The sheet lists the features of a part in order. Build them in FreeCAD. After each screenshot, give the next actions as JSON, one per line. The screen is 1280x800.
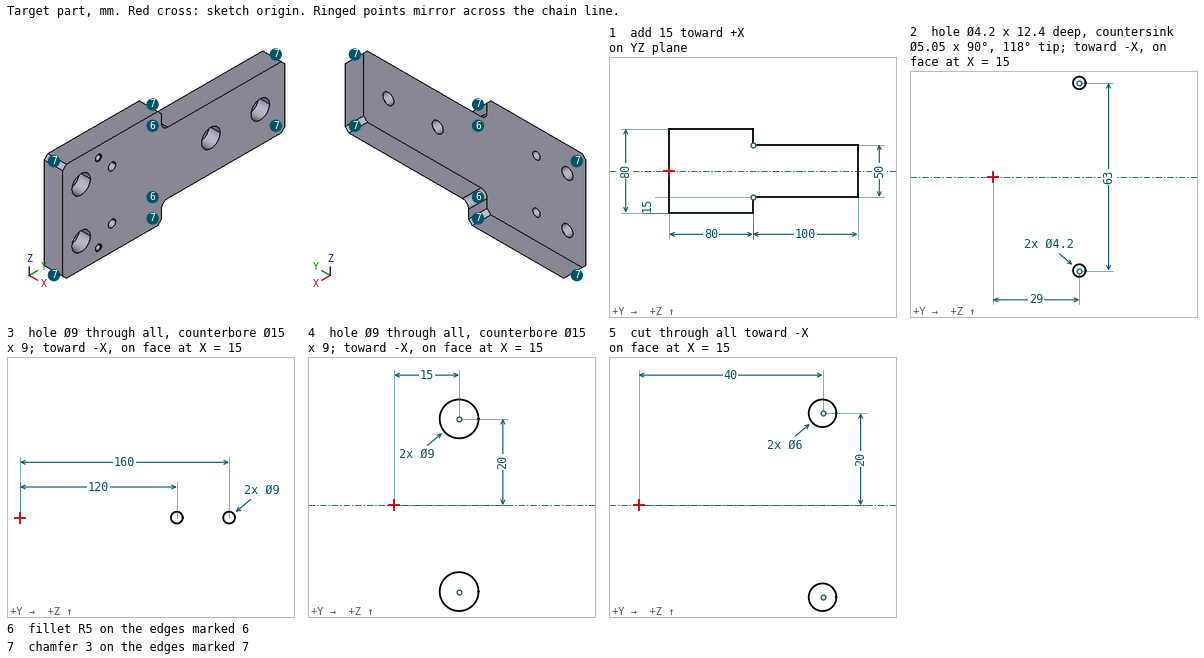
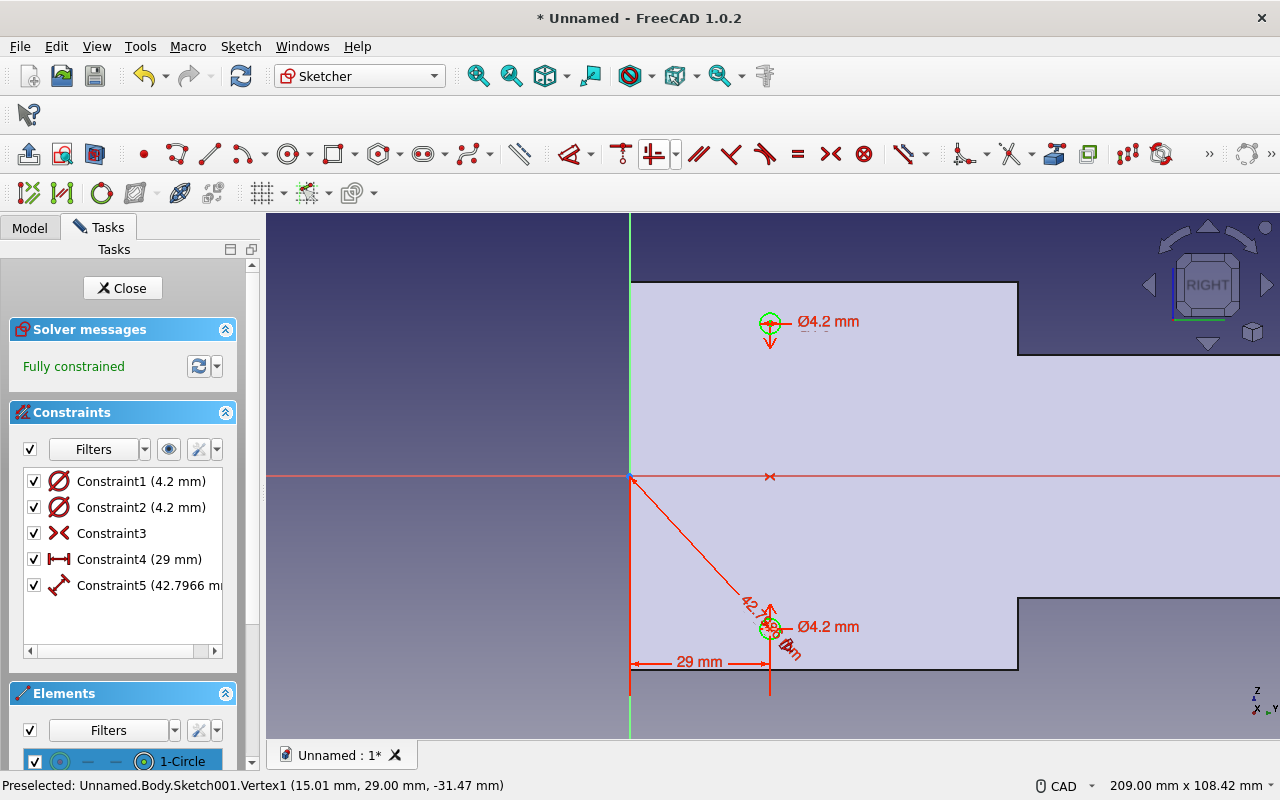
{"action": "left_click", "coordinate": [770, 324]}
{"action": "left_click", "coordinate": [804, 406]}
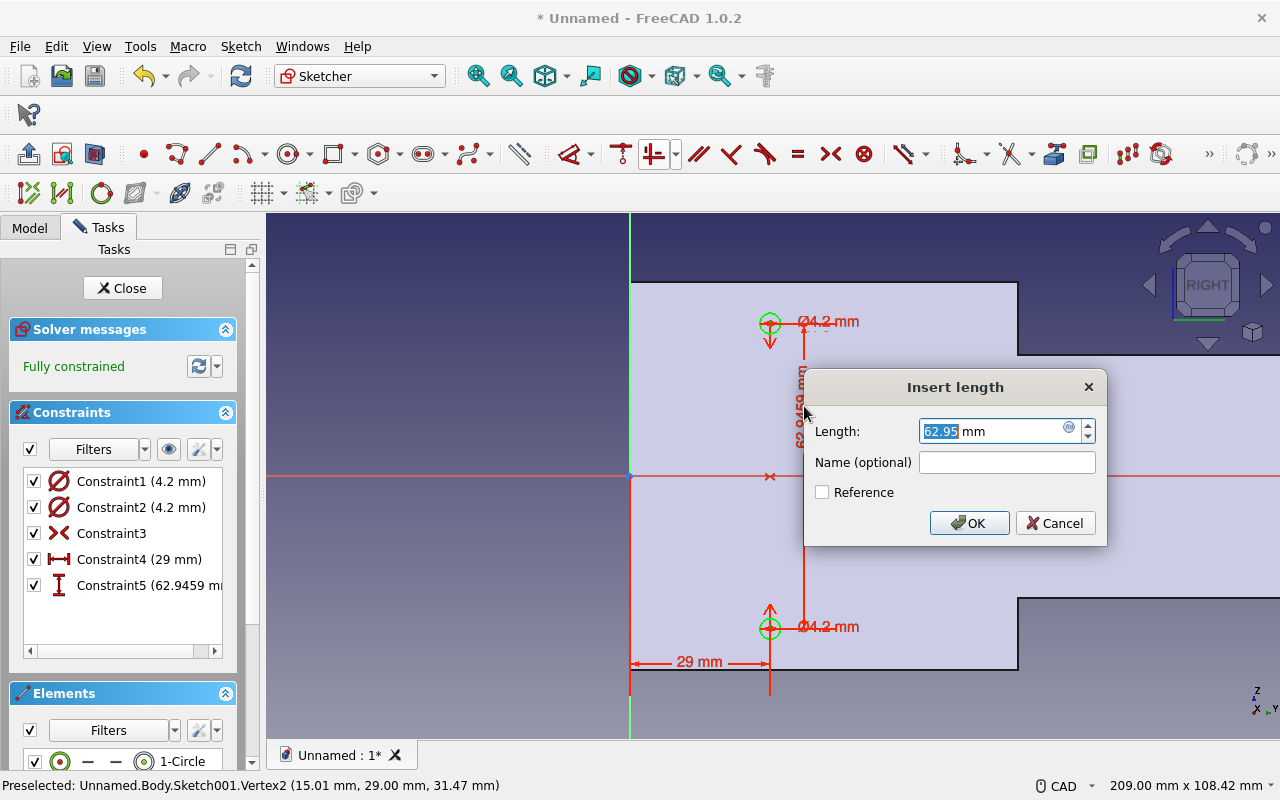
{"action": "type", "text": "63"}
{"action": "key", "text": "Return"}
{"action": "key", "text": "Escape"}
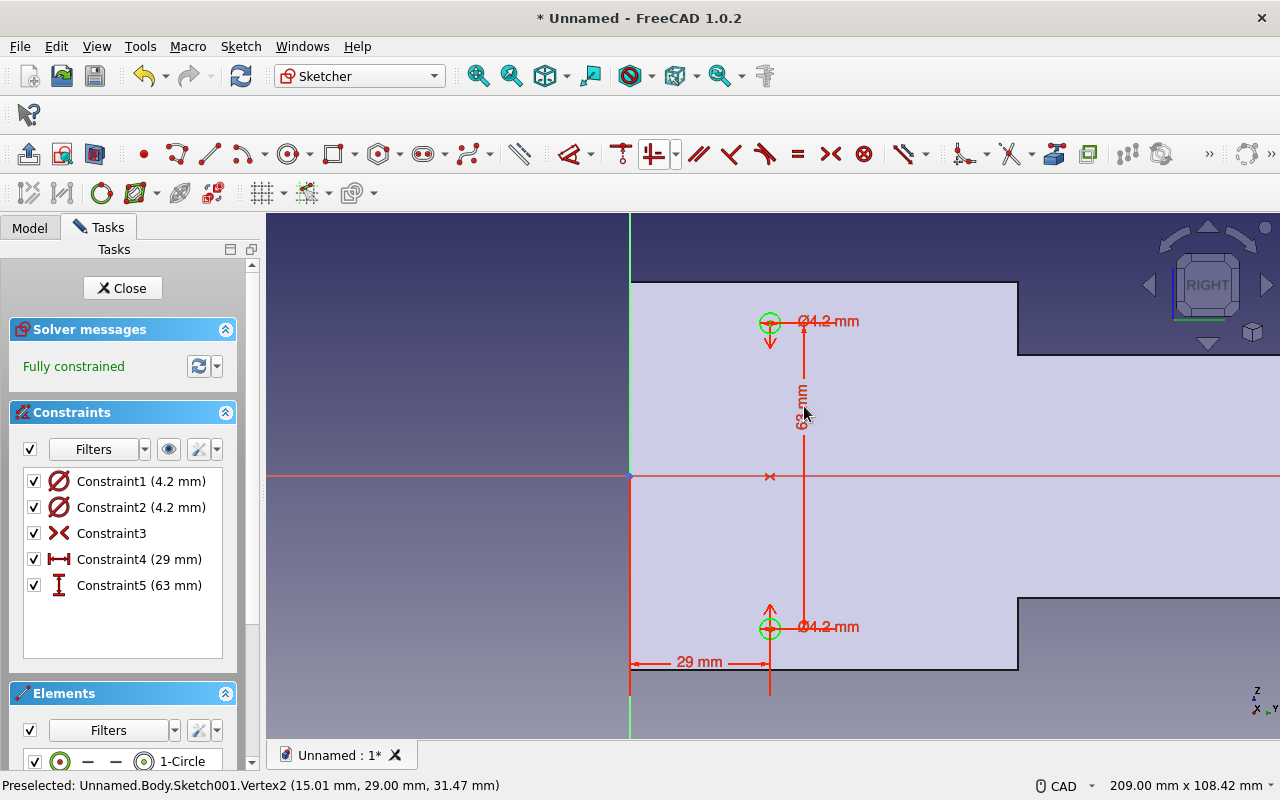
{"action": "left_click", "coordinate": [123, 288]}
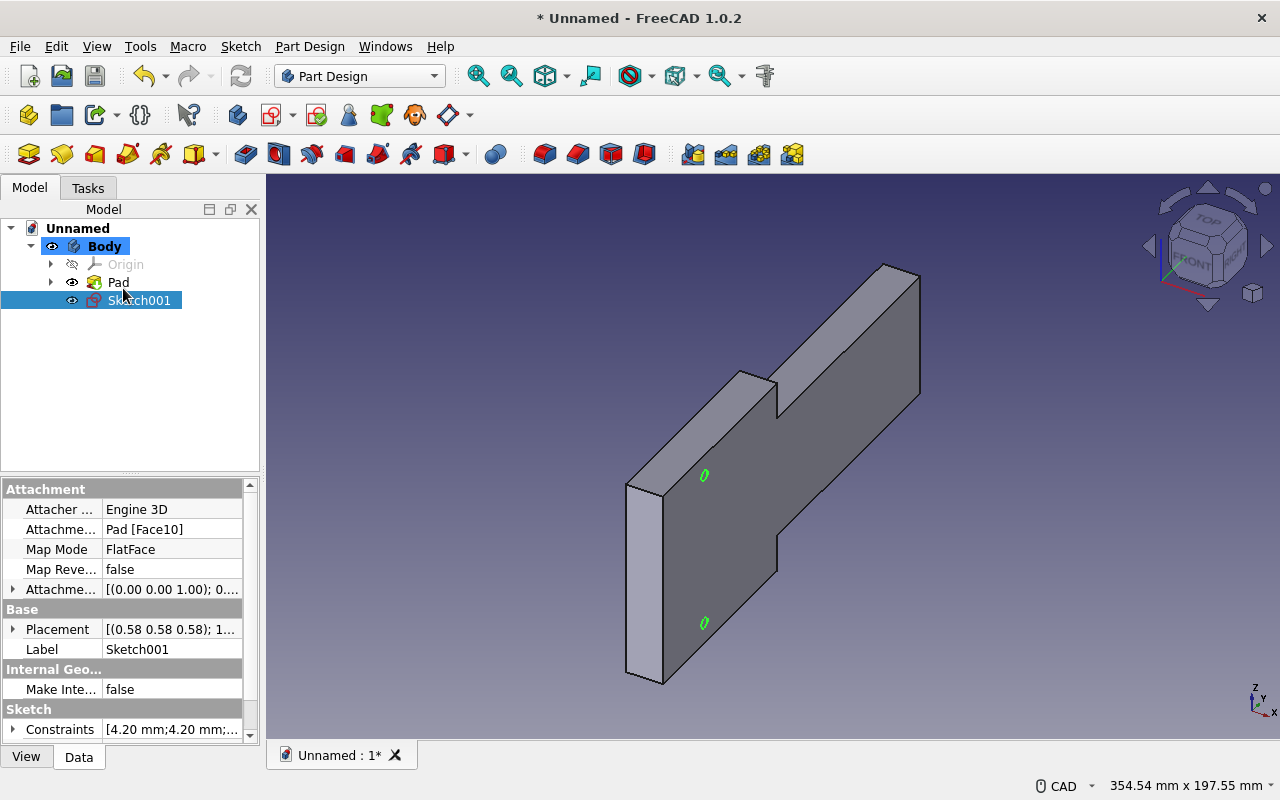
{"action": "left_click", "coordinate": [279, 154]}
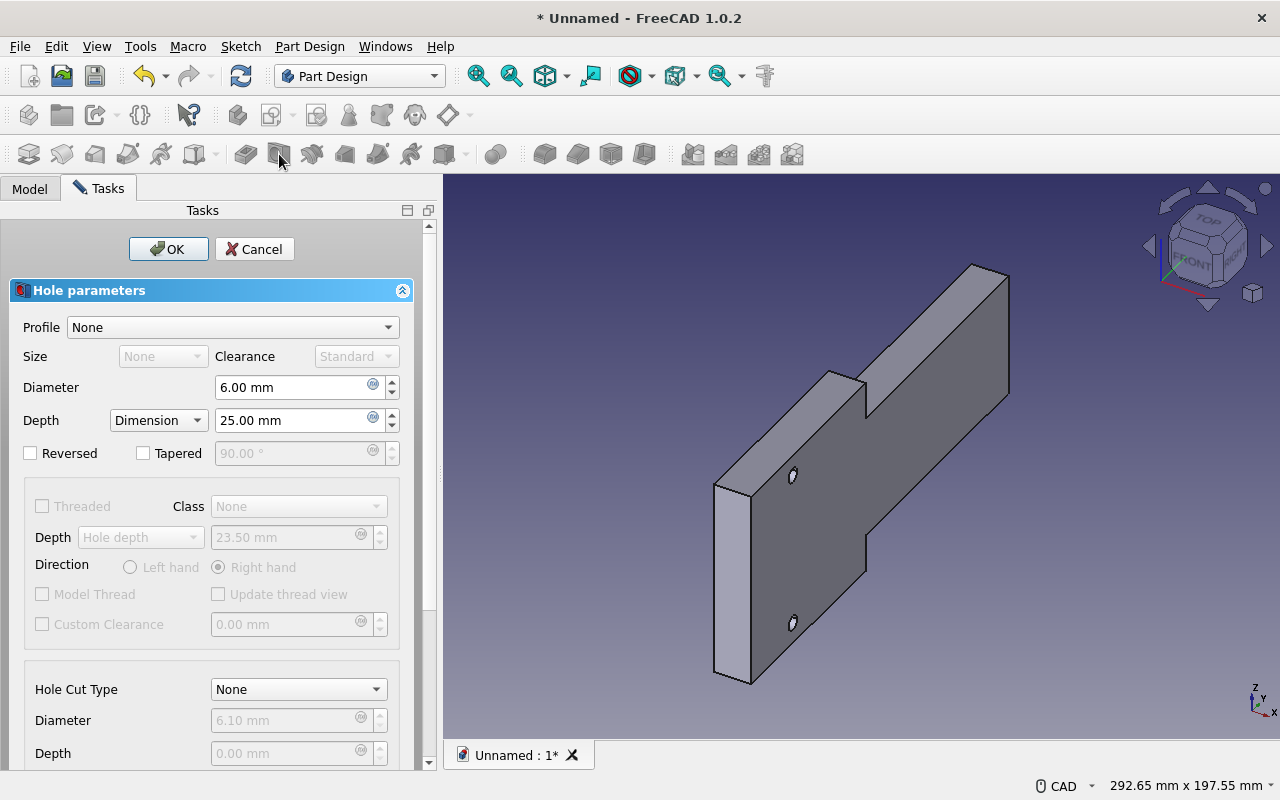
{"action": "triple_click", "coordinate": [300, 388]}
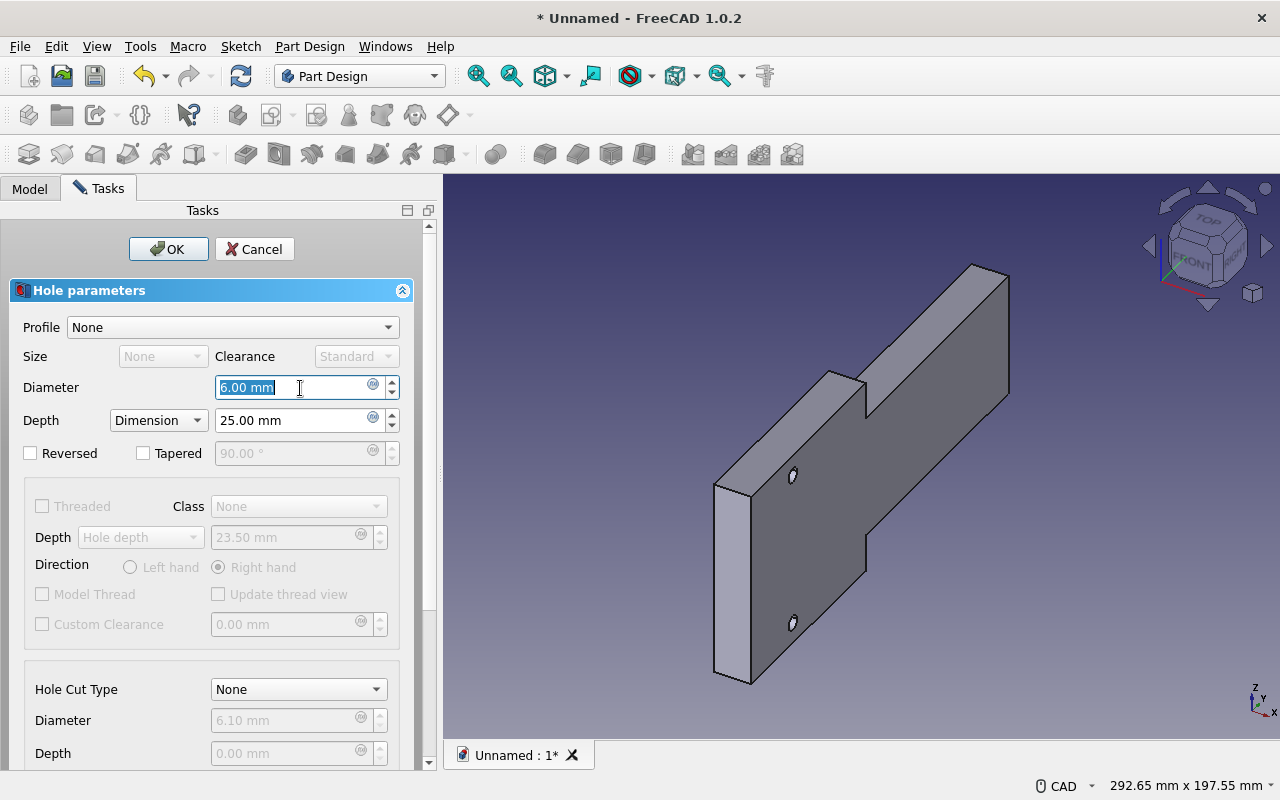
{"action": "type", "text": "4.2"}
{"action": "key", "text": "Tab"}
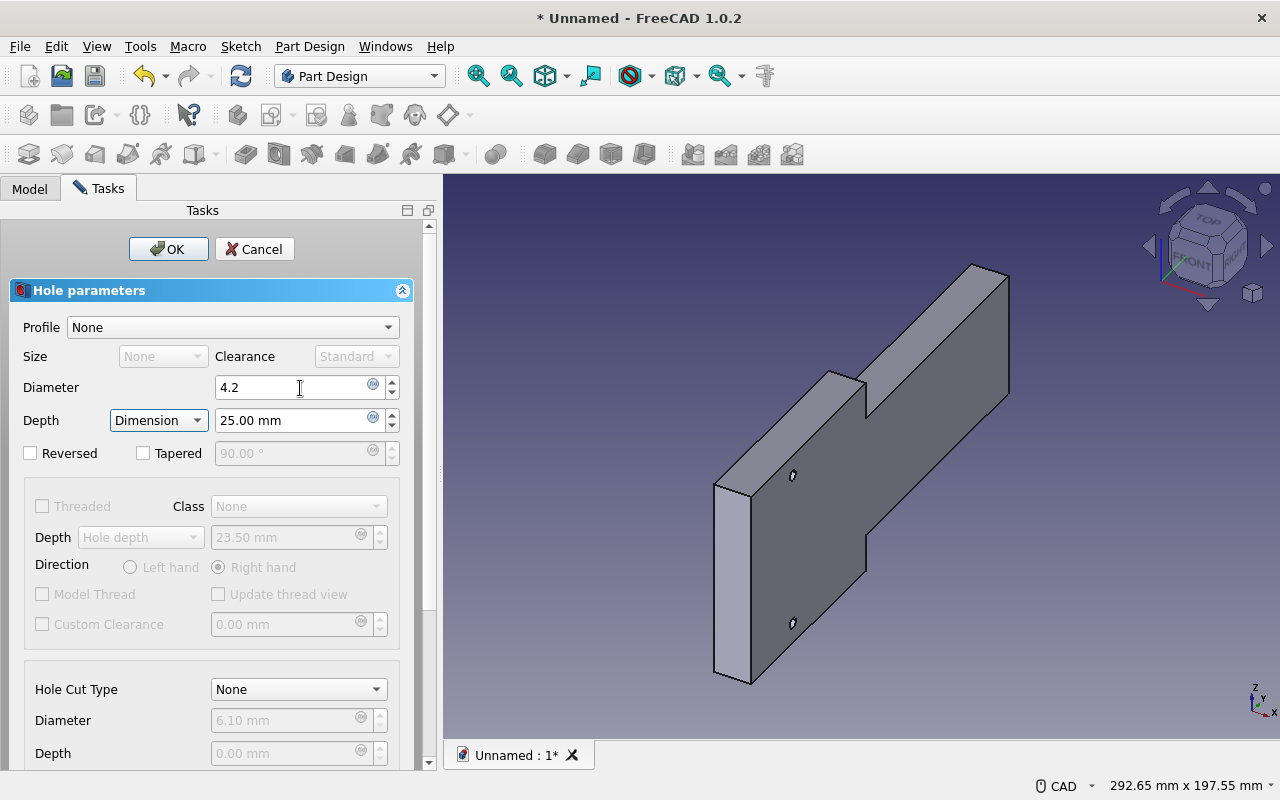
{"action": "triple_click", "coordinate": [300, 420]}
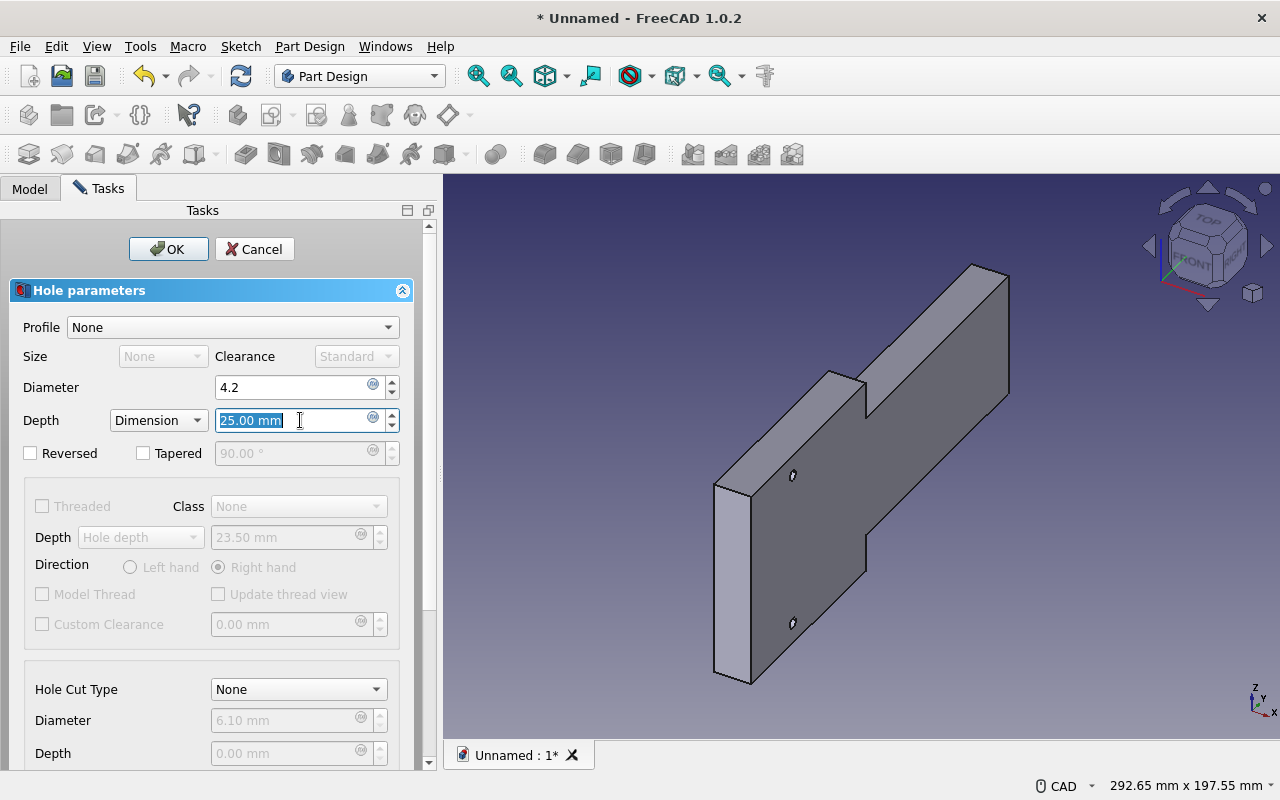
{"action": "type", "text": "12.4"}
{"action": "key", "text": "Tab"}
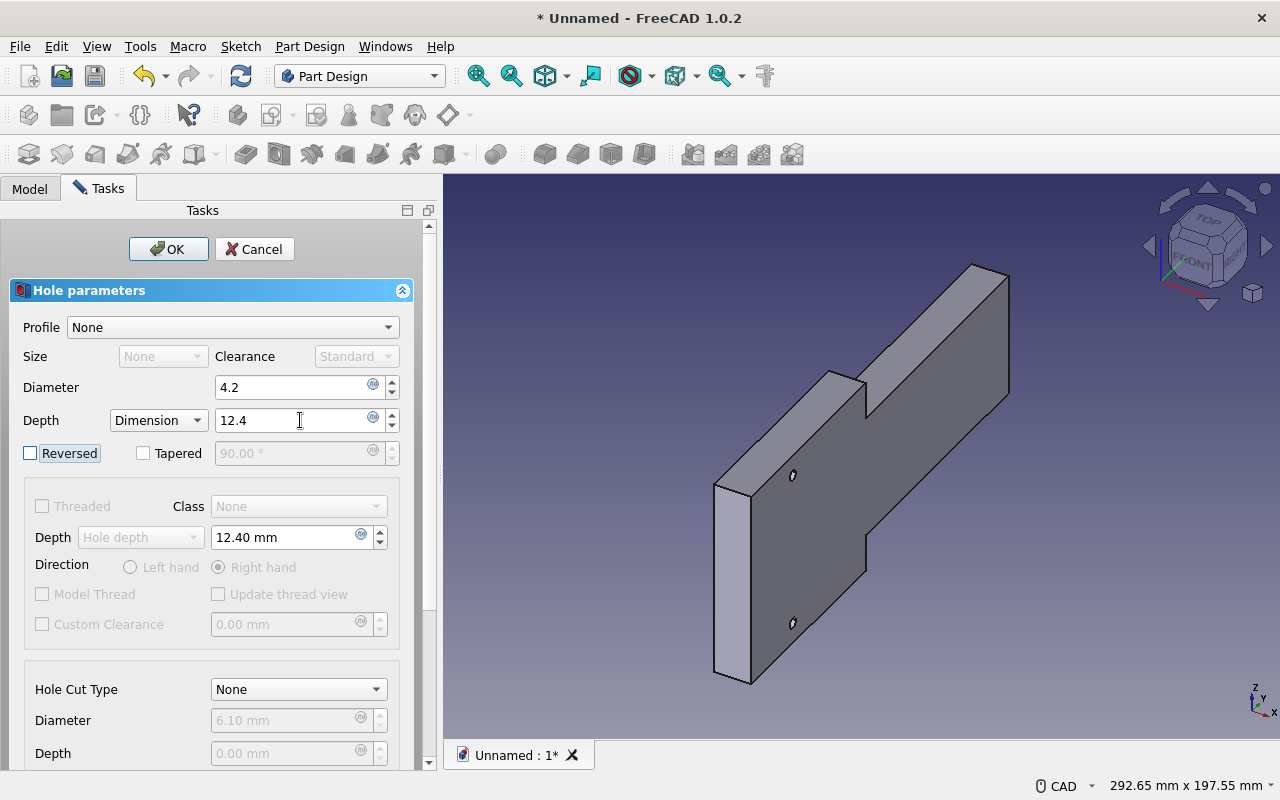
{"action": "left_click", "coordinate": [300, 690]}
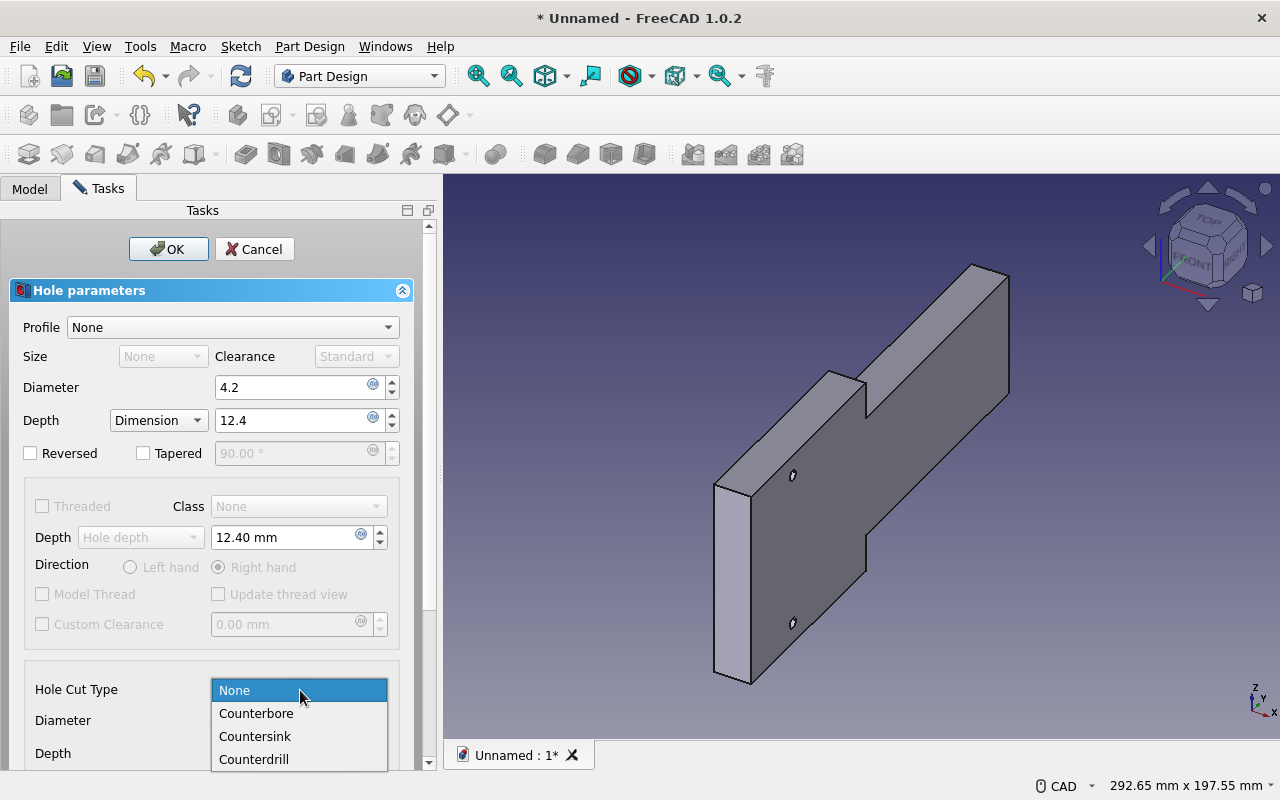
{"action": "left_click", "coordinate": [298, 736]}